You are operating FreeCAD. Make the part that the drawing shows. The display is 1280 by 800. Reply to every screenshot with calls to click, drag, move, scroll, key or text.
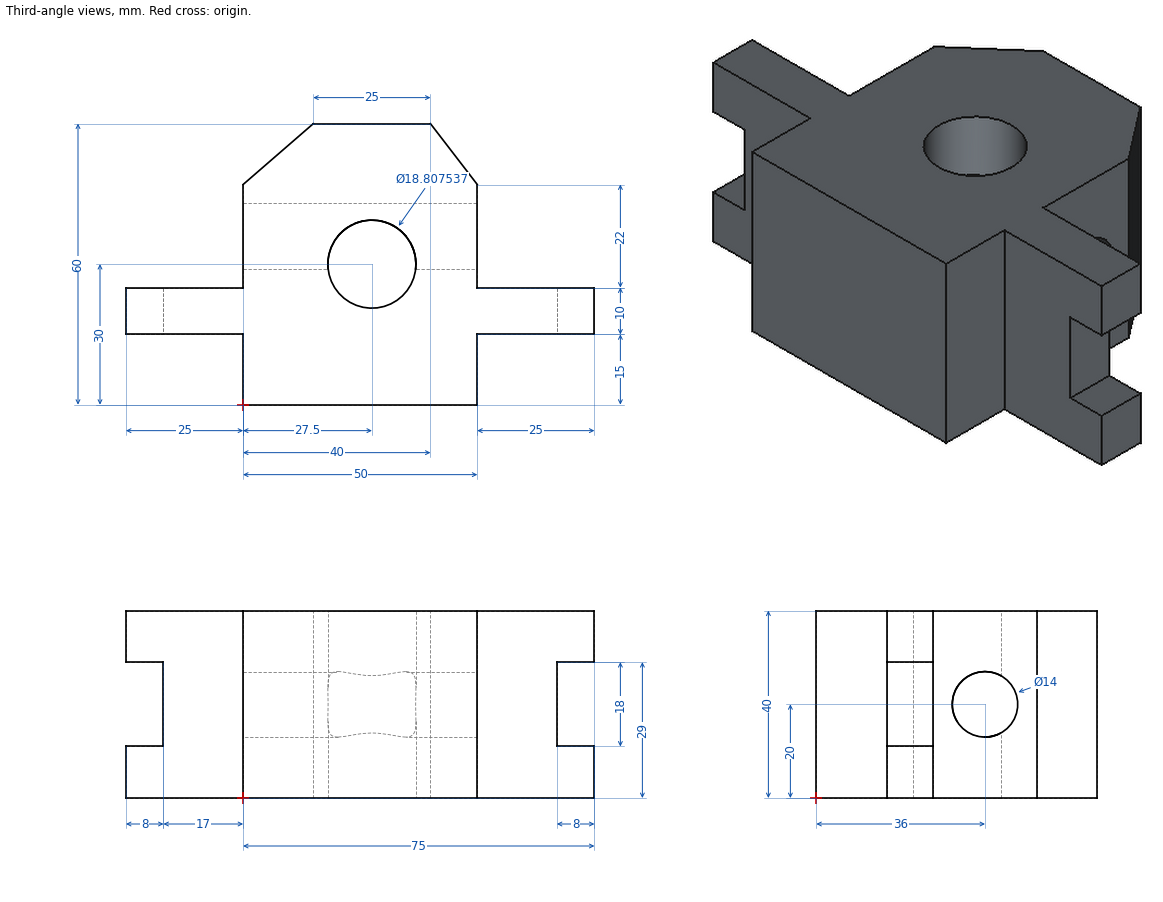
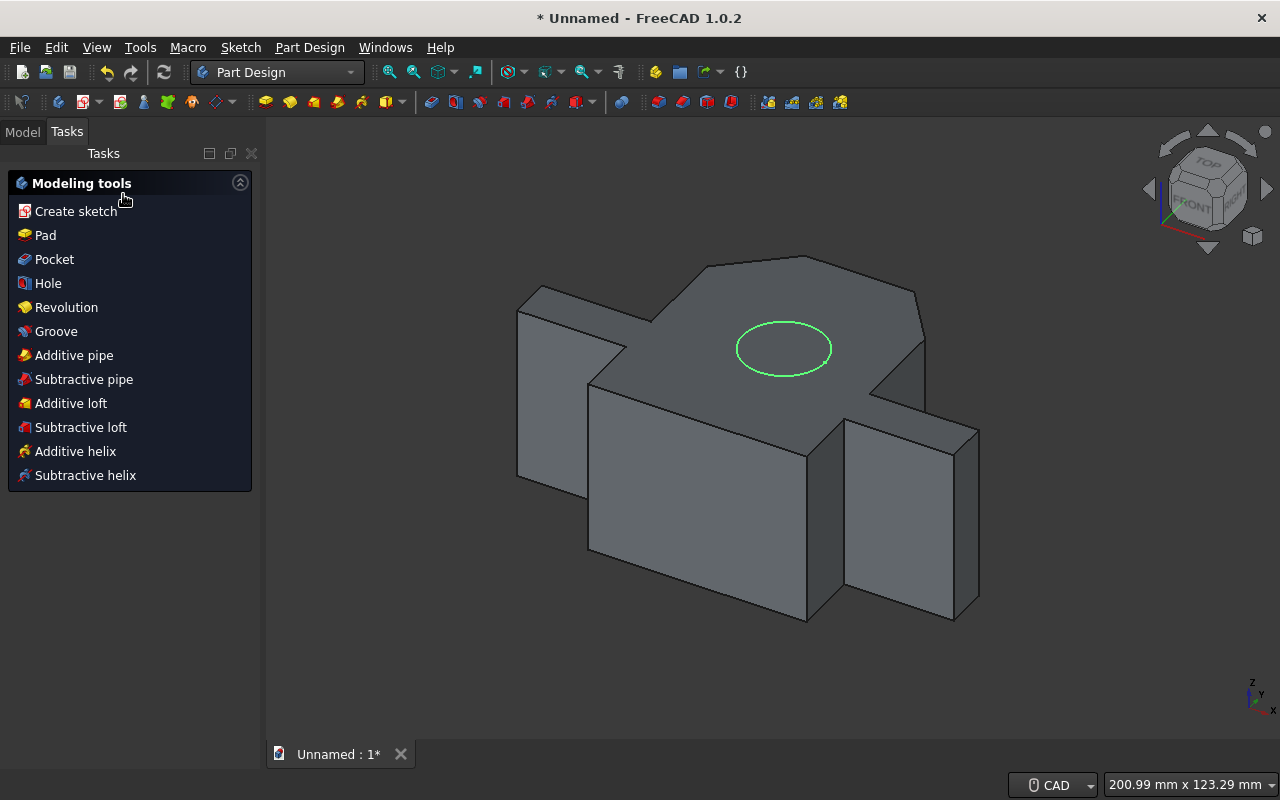
click(432, 102)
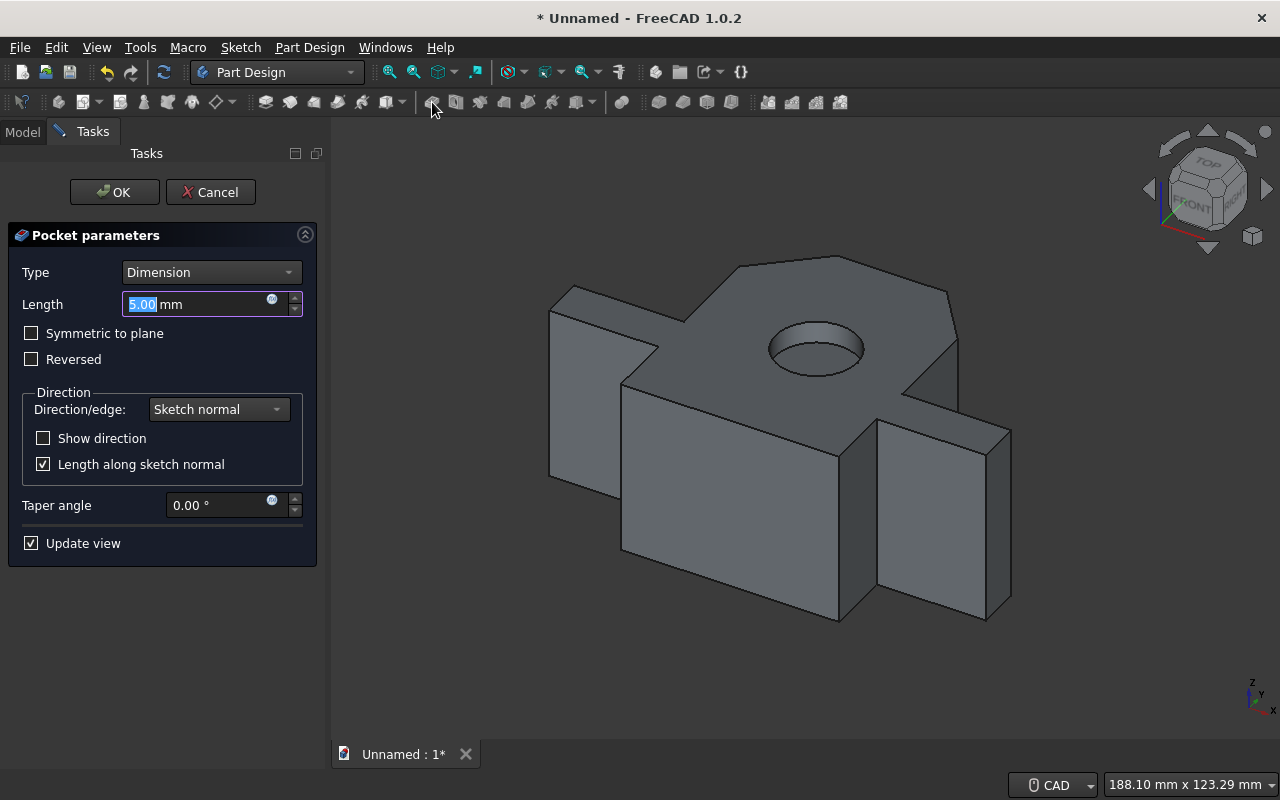
click(212, 272)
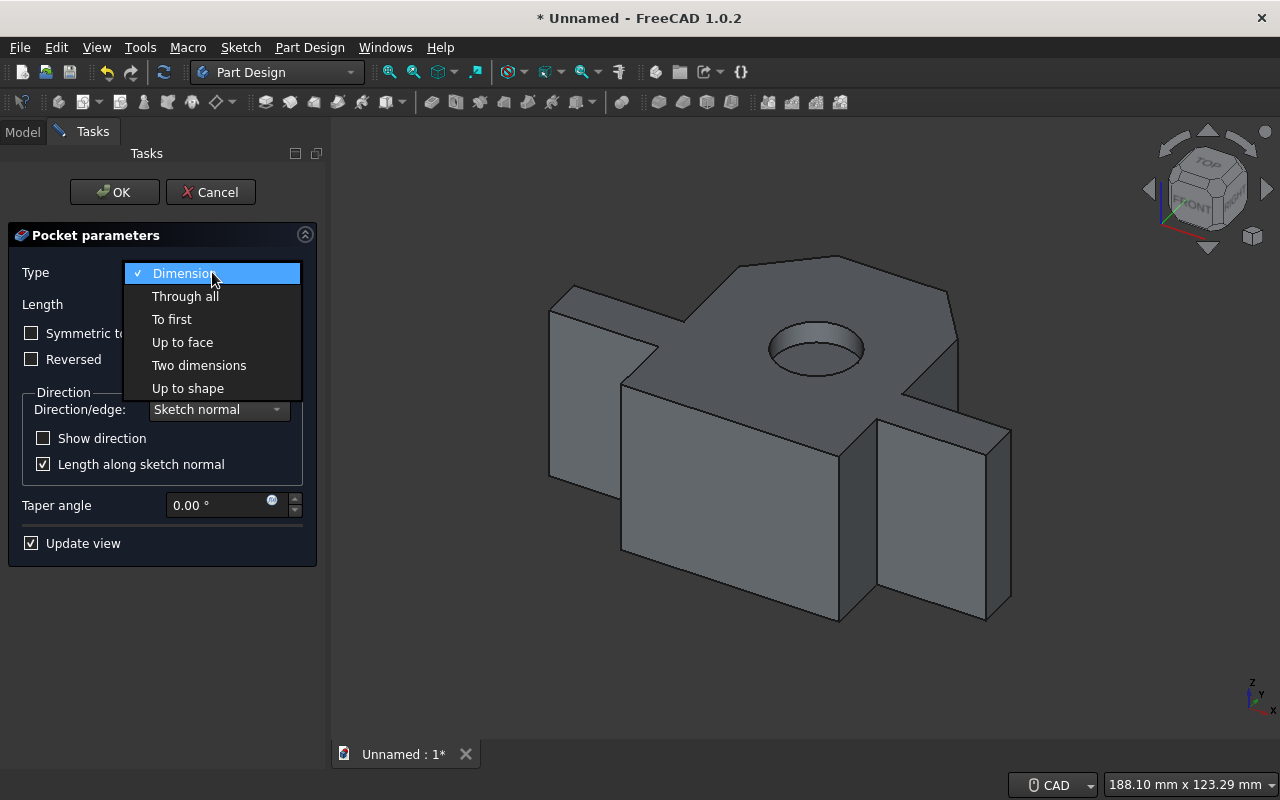
click(212, 296)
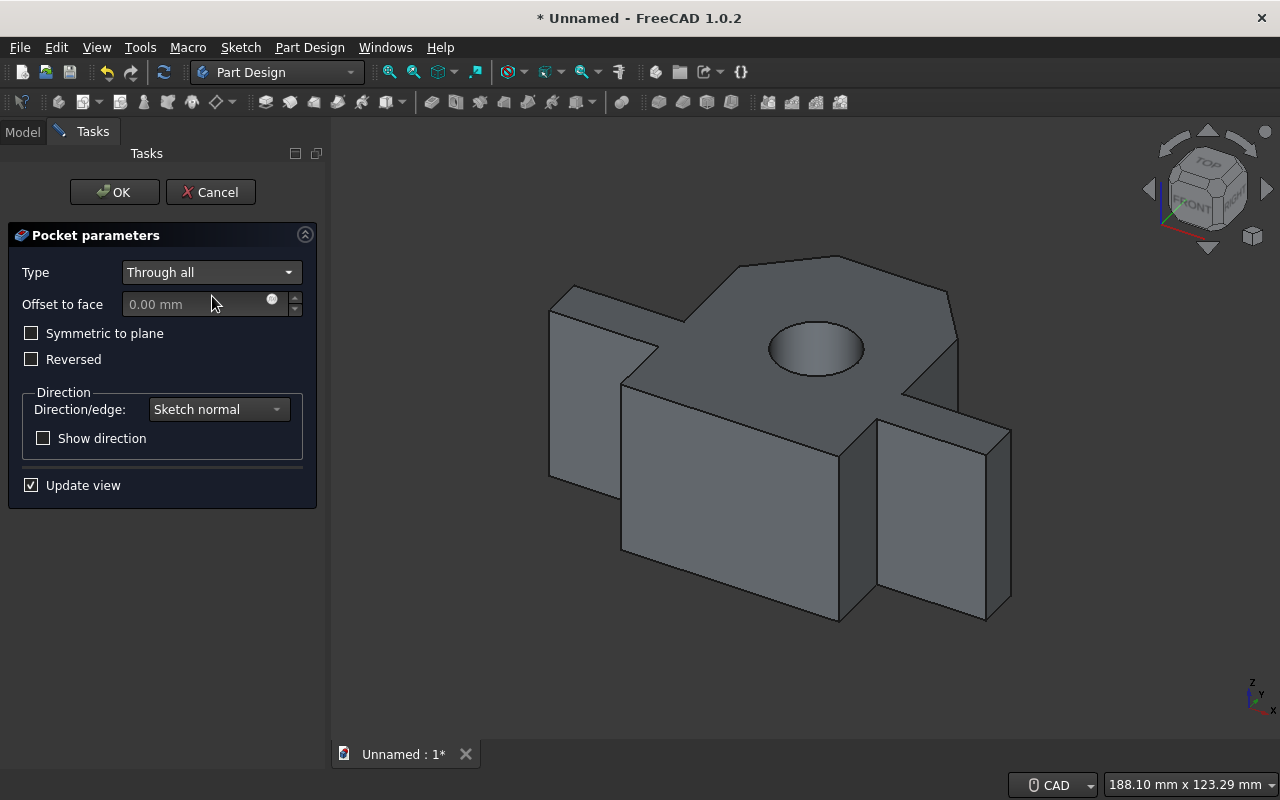
click(115, 192)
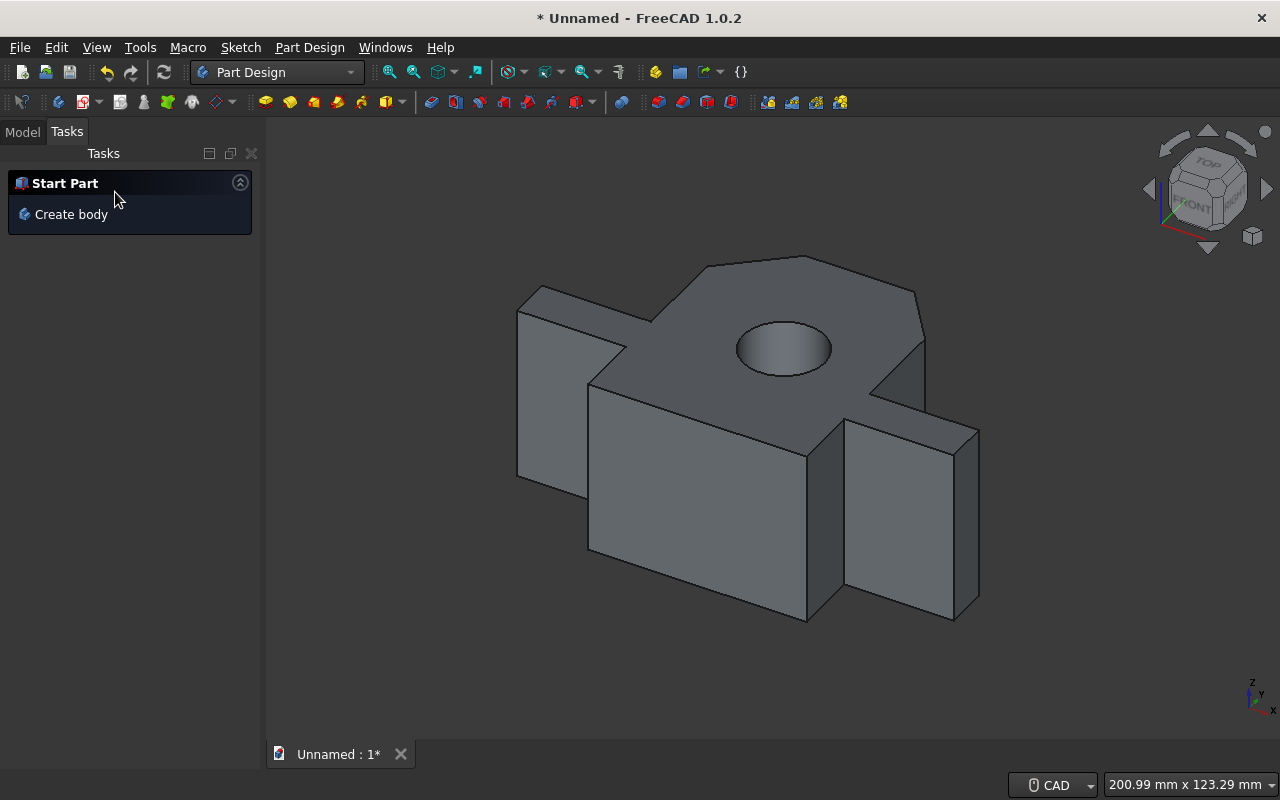
key(4)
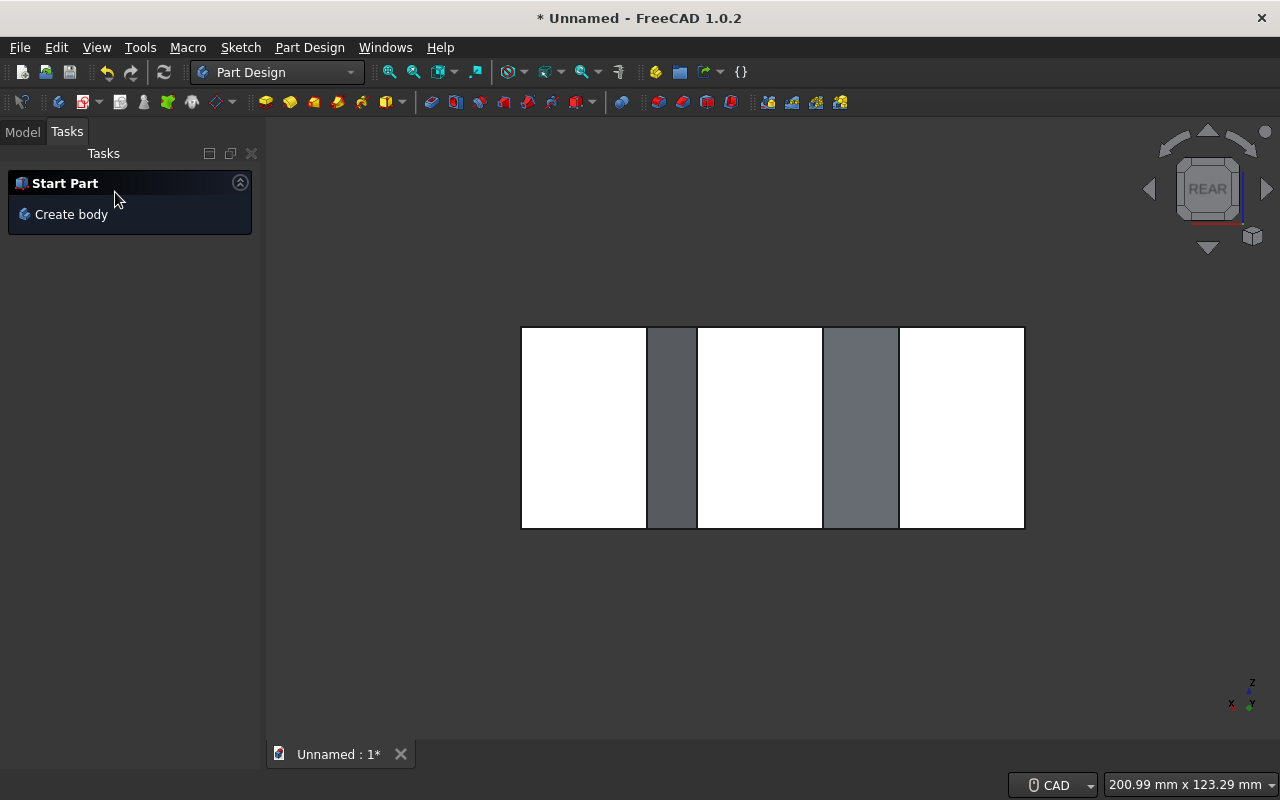
click(584, 398)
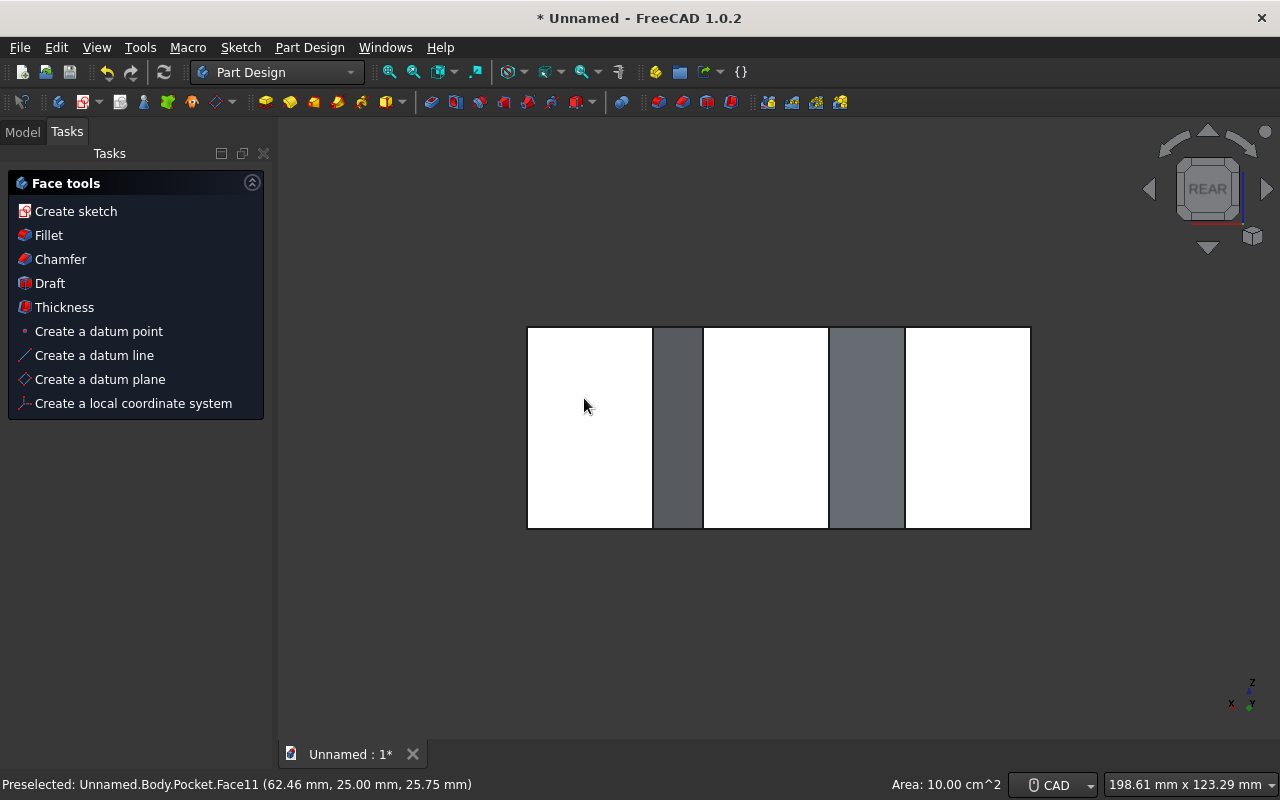
click(84, 102)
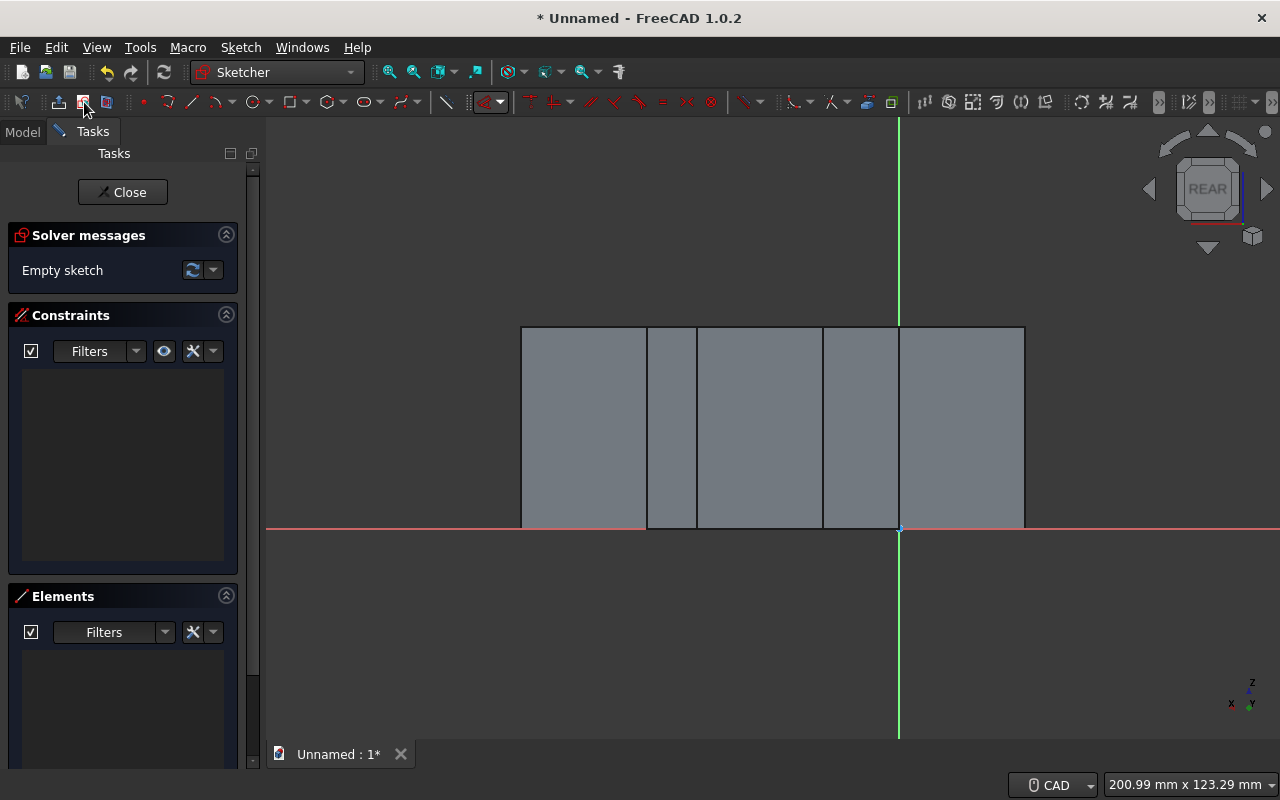
key(q)
key(s)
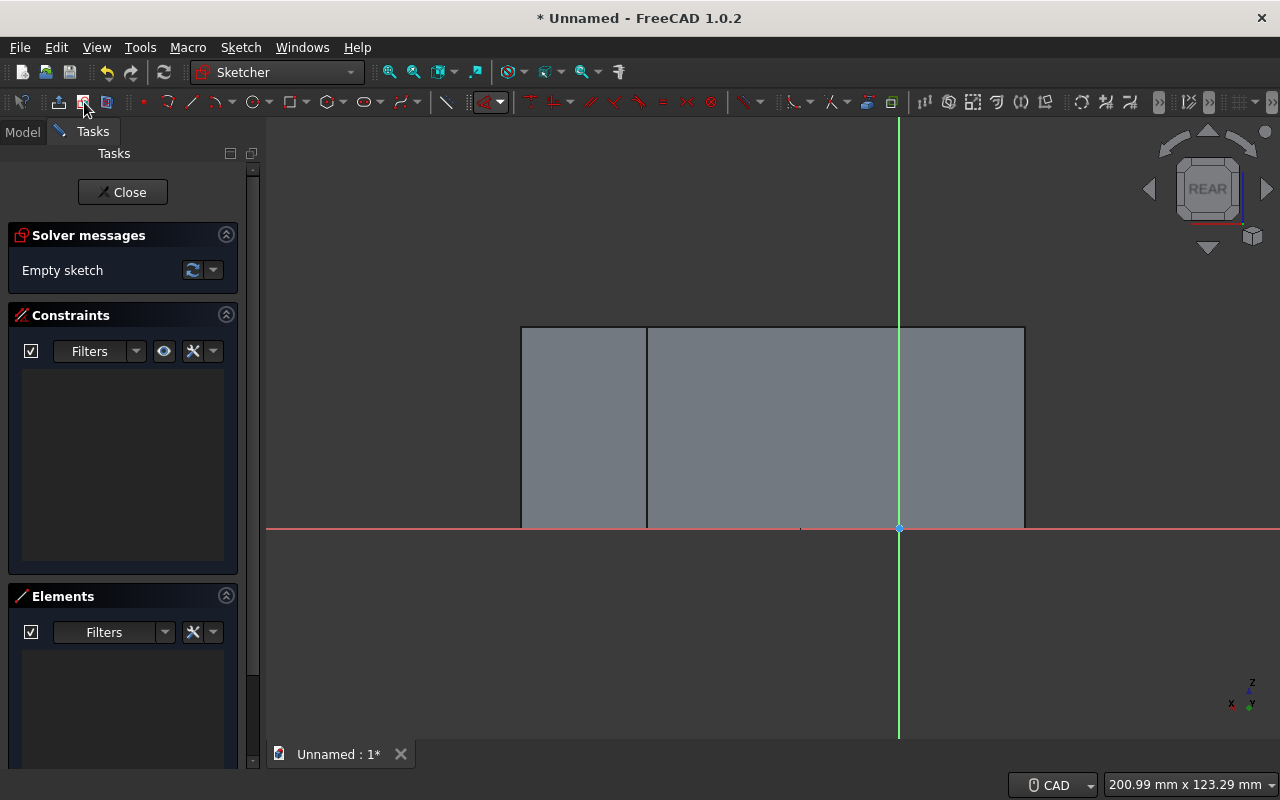
scroll(487, 428, up, 7)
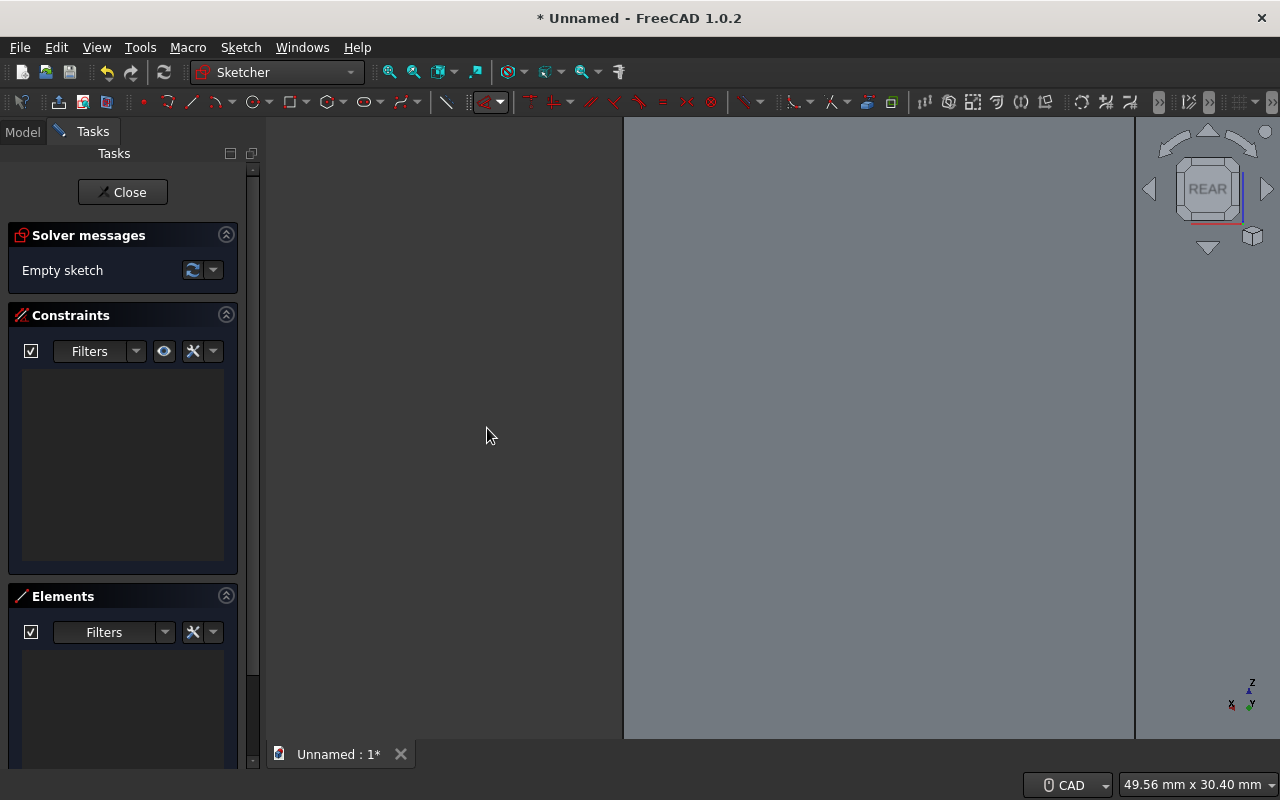
key(g)
key(r)